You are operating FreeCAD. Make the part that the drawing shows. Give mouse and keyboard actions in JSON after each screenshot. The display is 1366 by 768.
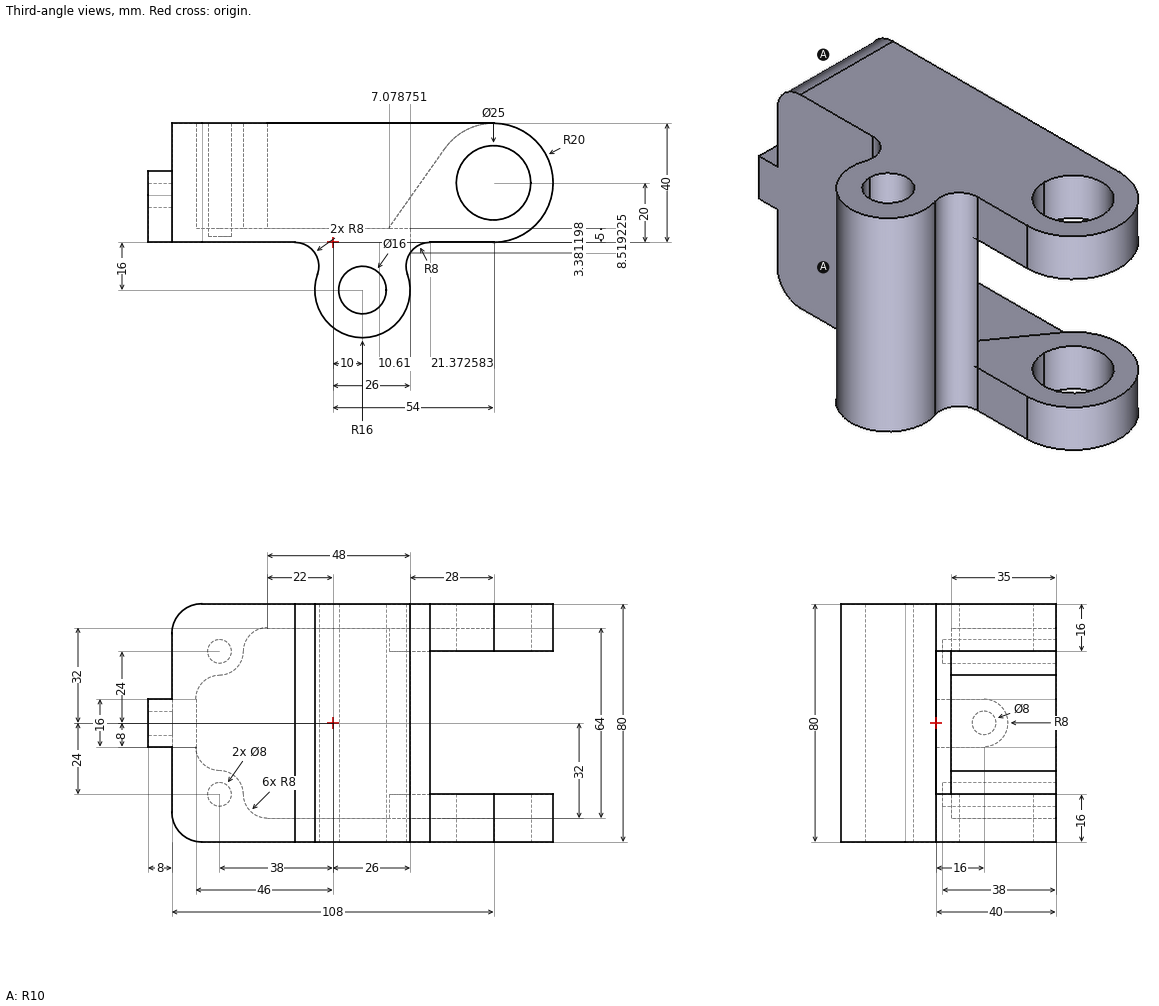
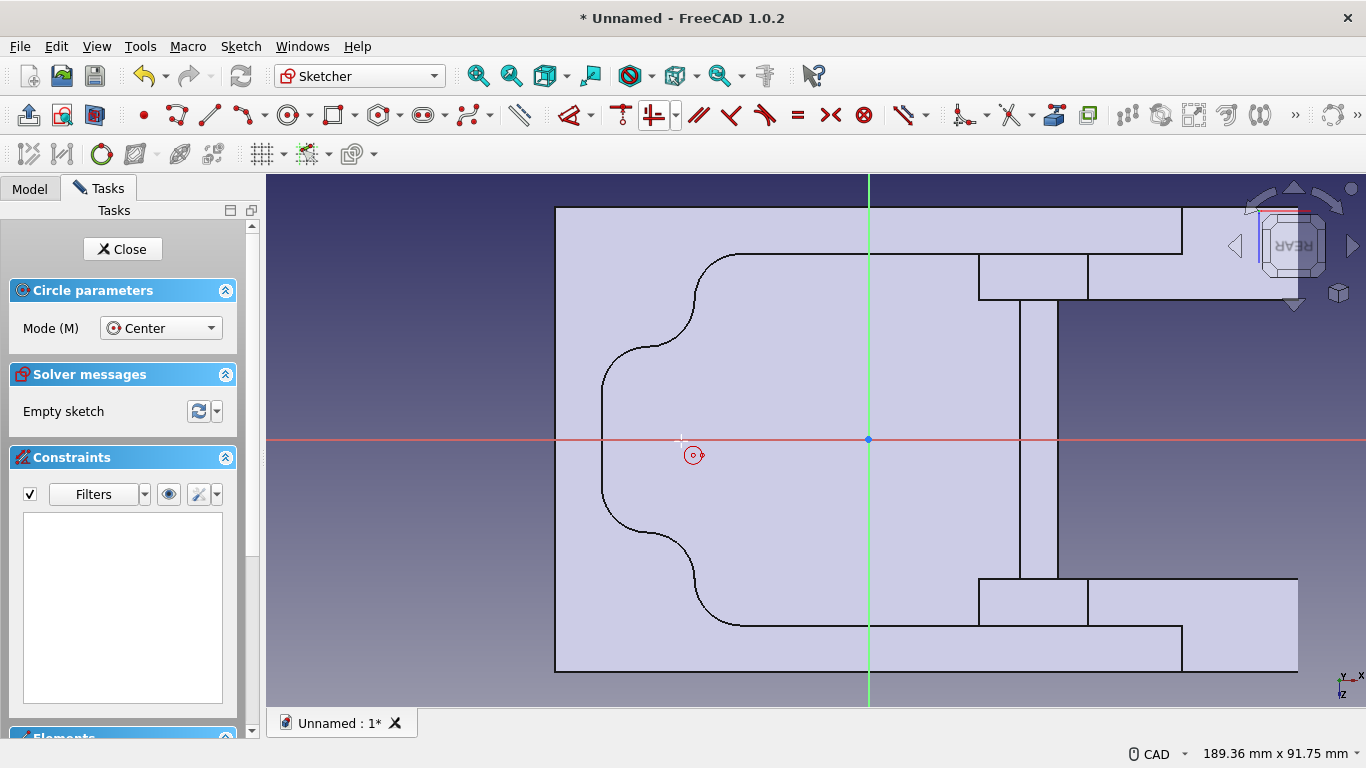
{"action": "left_click", "coordinate": [648, 300]}
{"action": "mouse_move", "coordinate": [664, 284]}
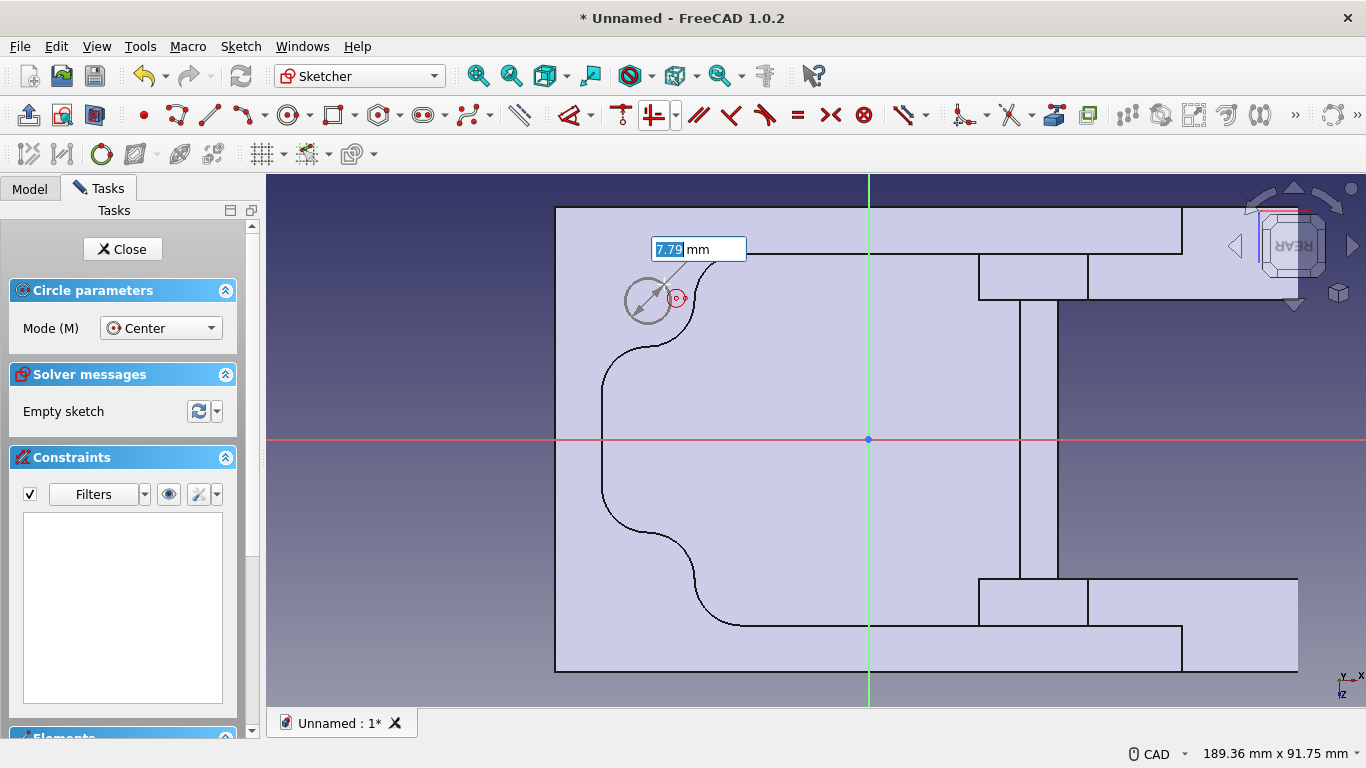
{"action": "type", "text": "8"}
{"action": "key", "text": "Return"}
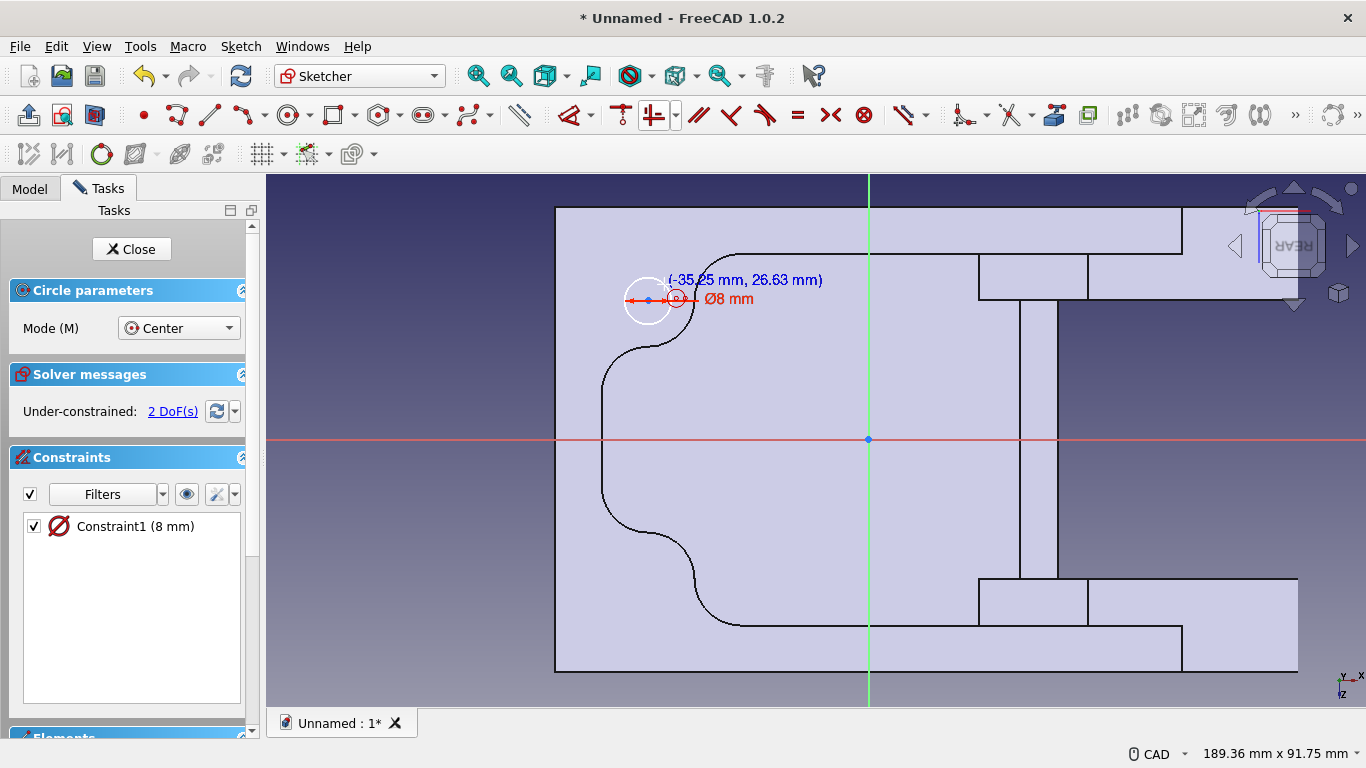
{"action": "left_click", "coordinate": [648, 579]}
{"action": "mouse_move", "coordinate": [664, 563]}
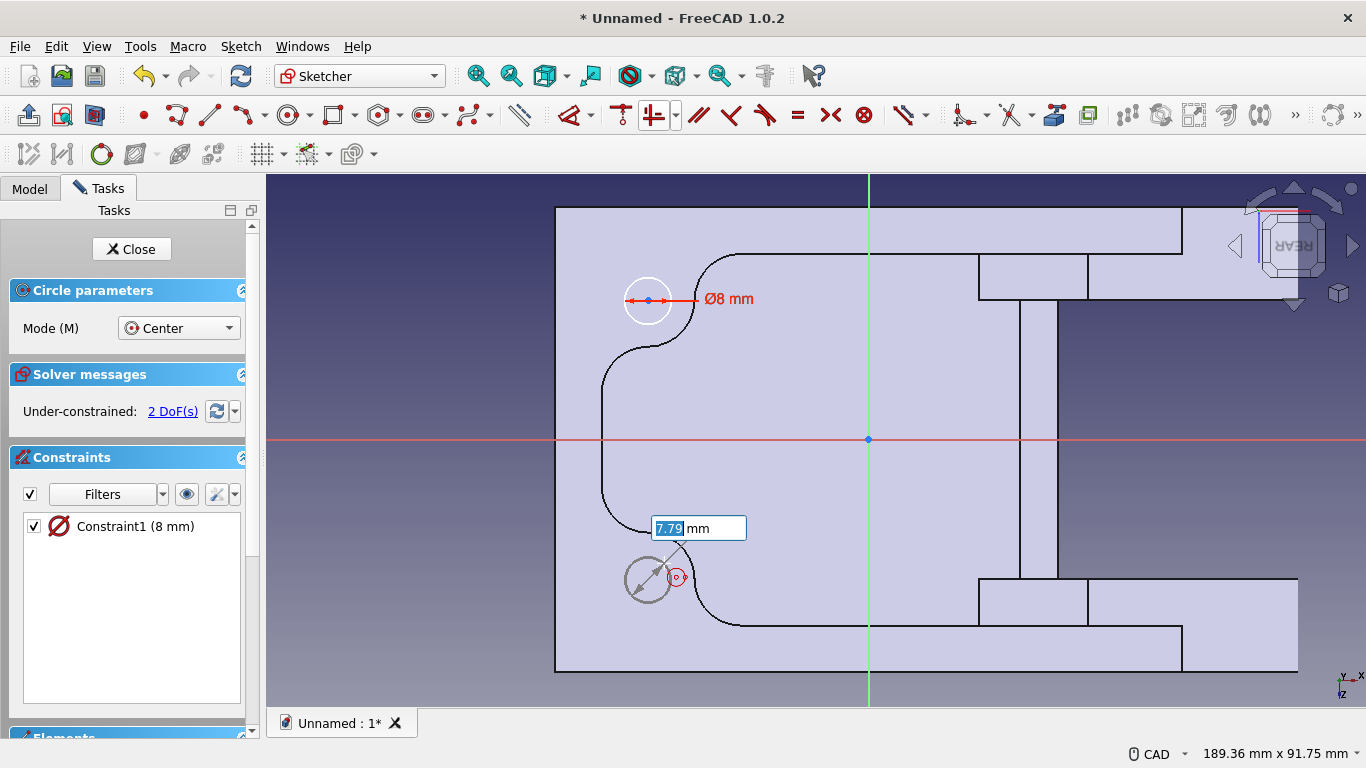
{"action": "type", "text": "8"}
{"action": "key", "text": "Return"}
{"action": "key", "text": "Escape"}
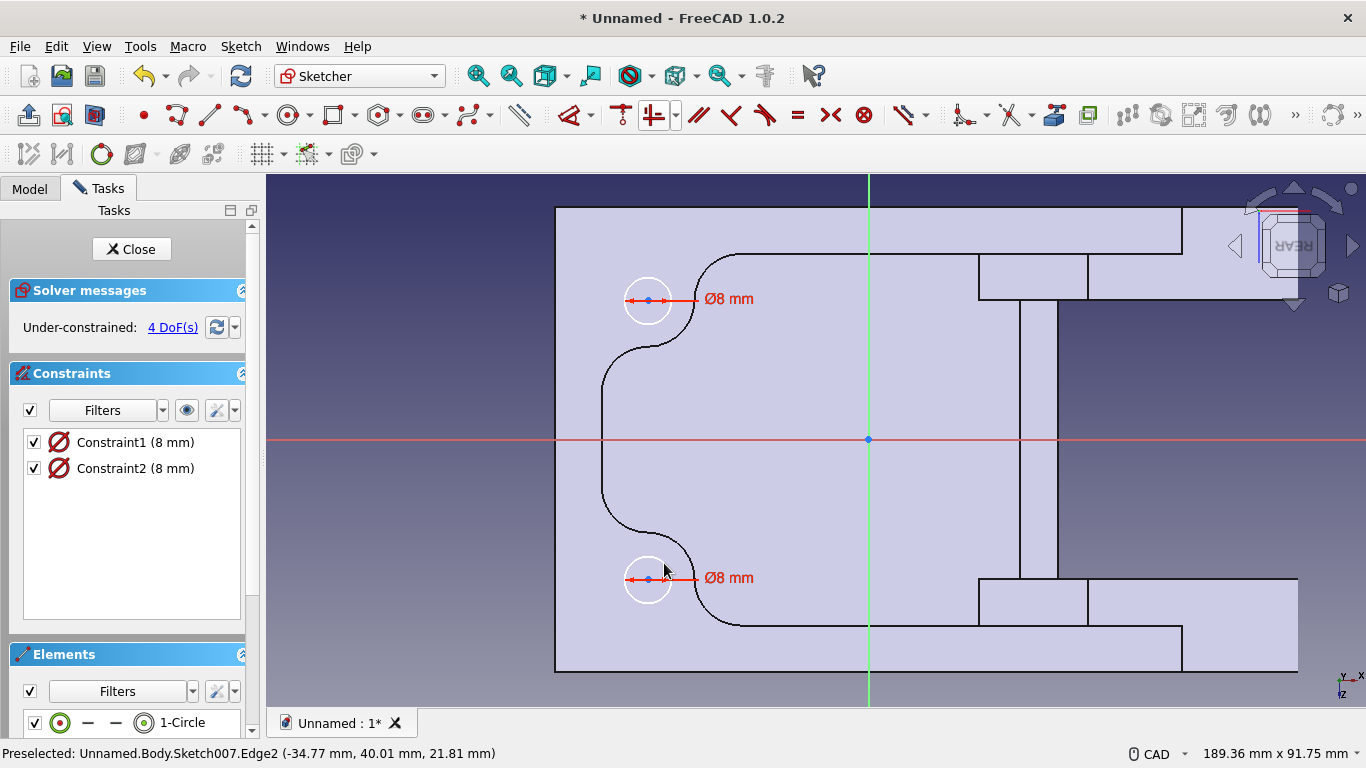
{"action": "left_click", "coordinate": [648, 301]}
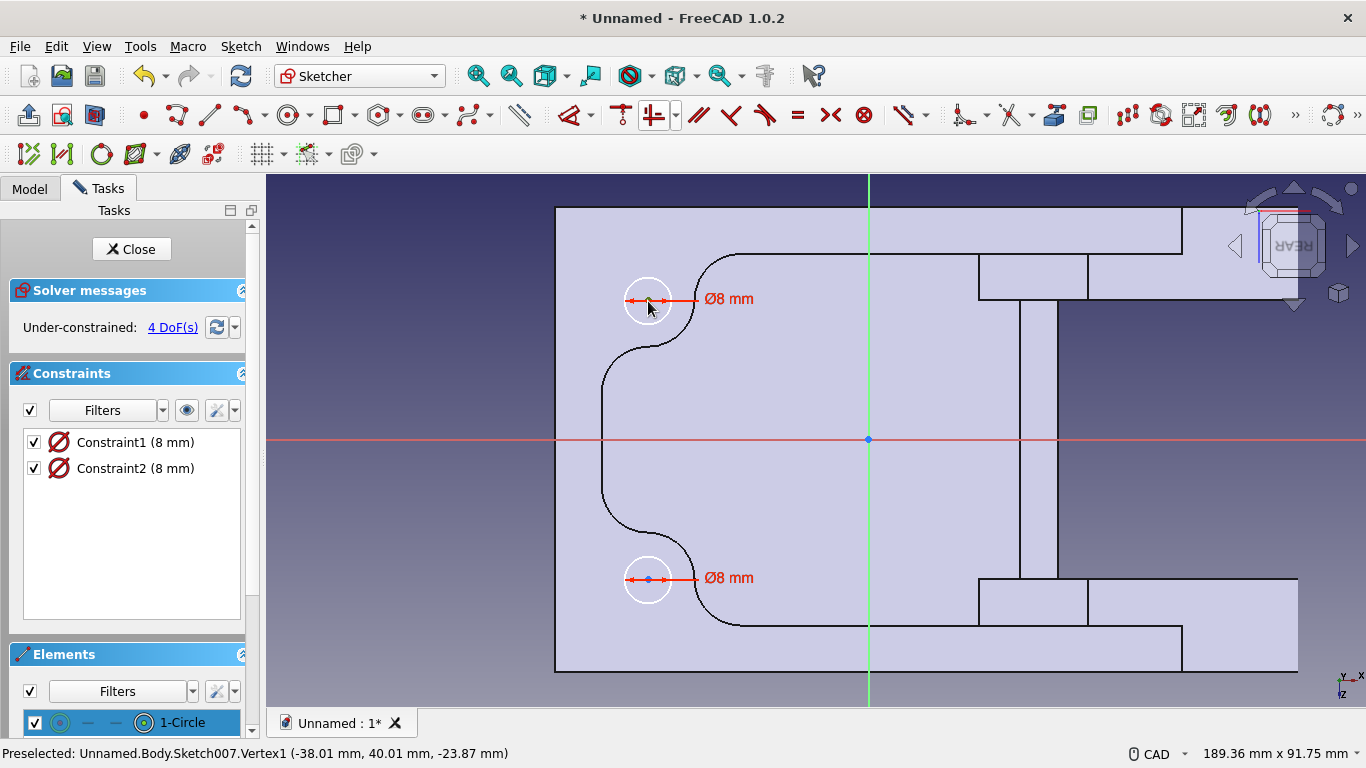
{"action": "left_click", "coordinate": [648, 580]}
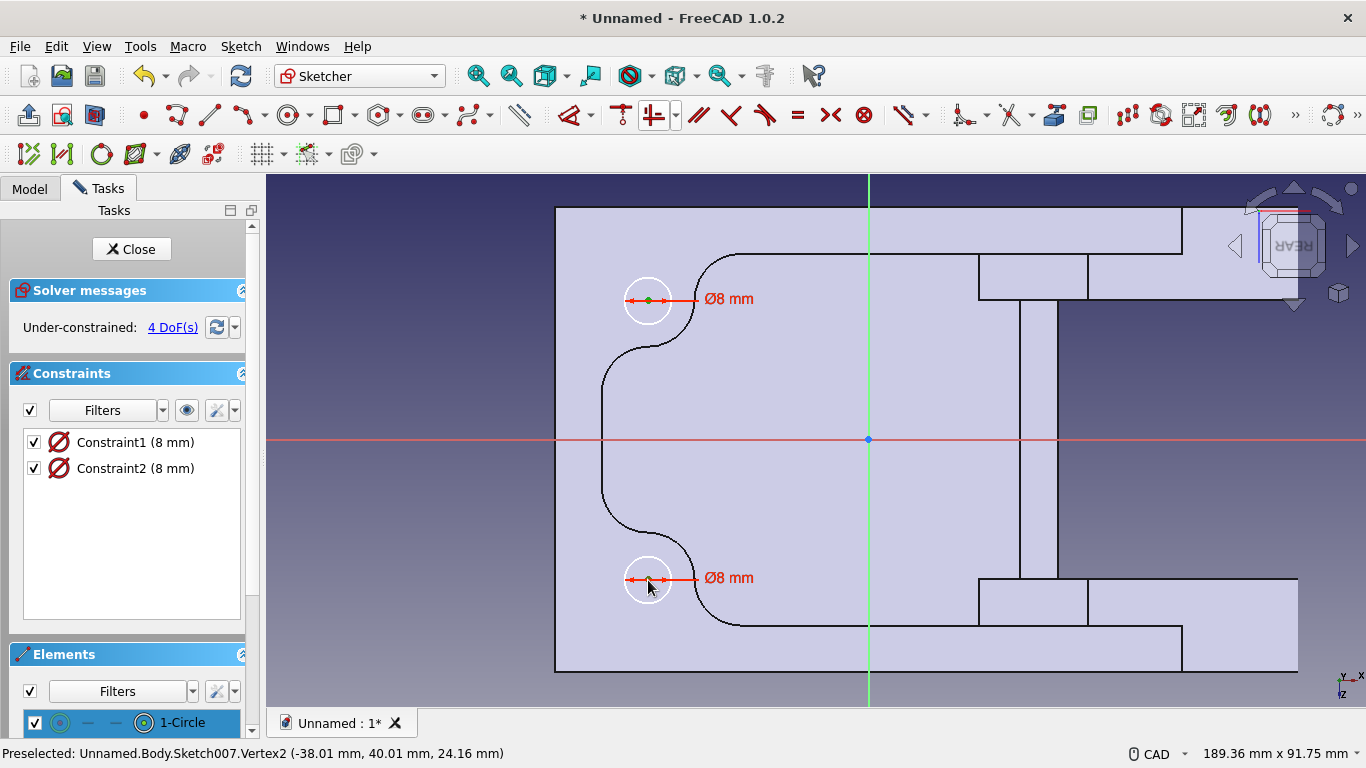
{"action": "left_click", "coordinate": [676, 116]}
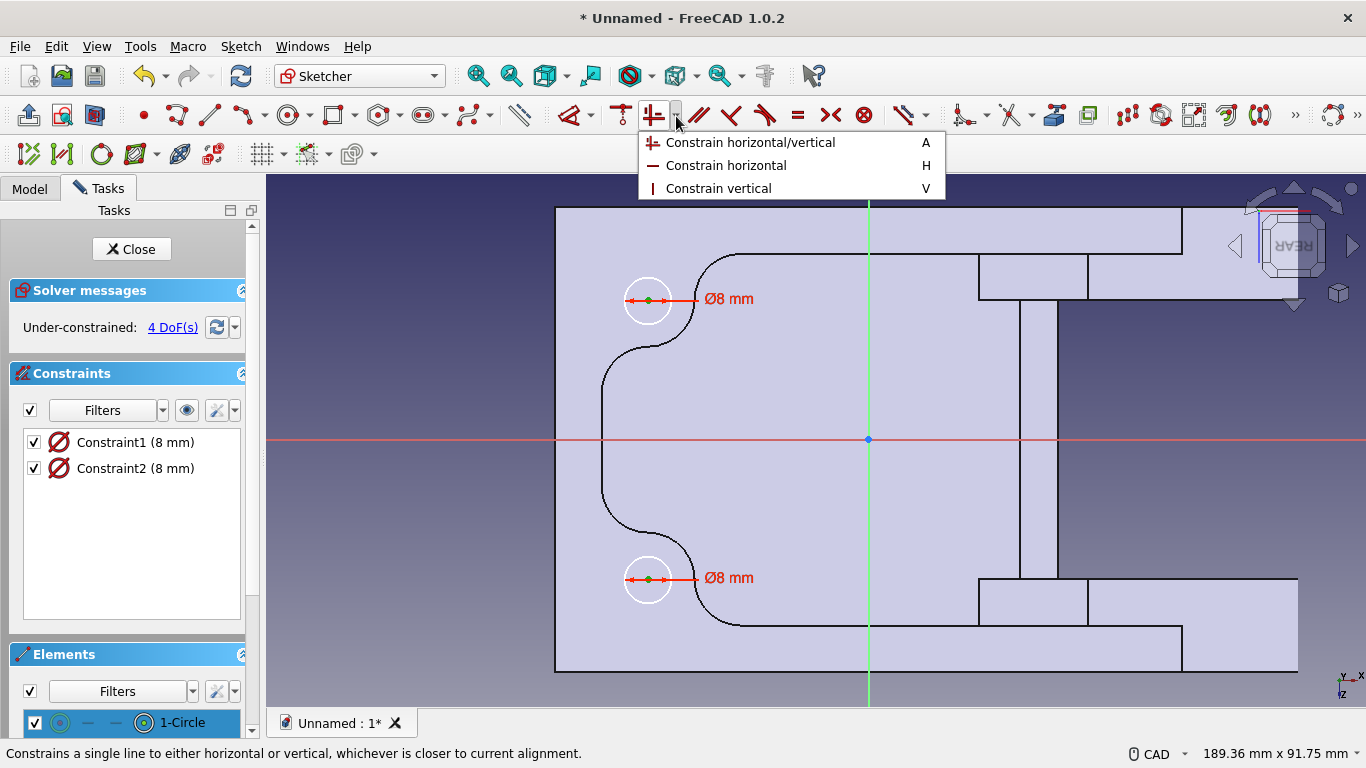
{"action": "left_click", "coordinate": [792, 188]}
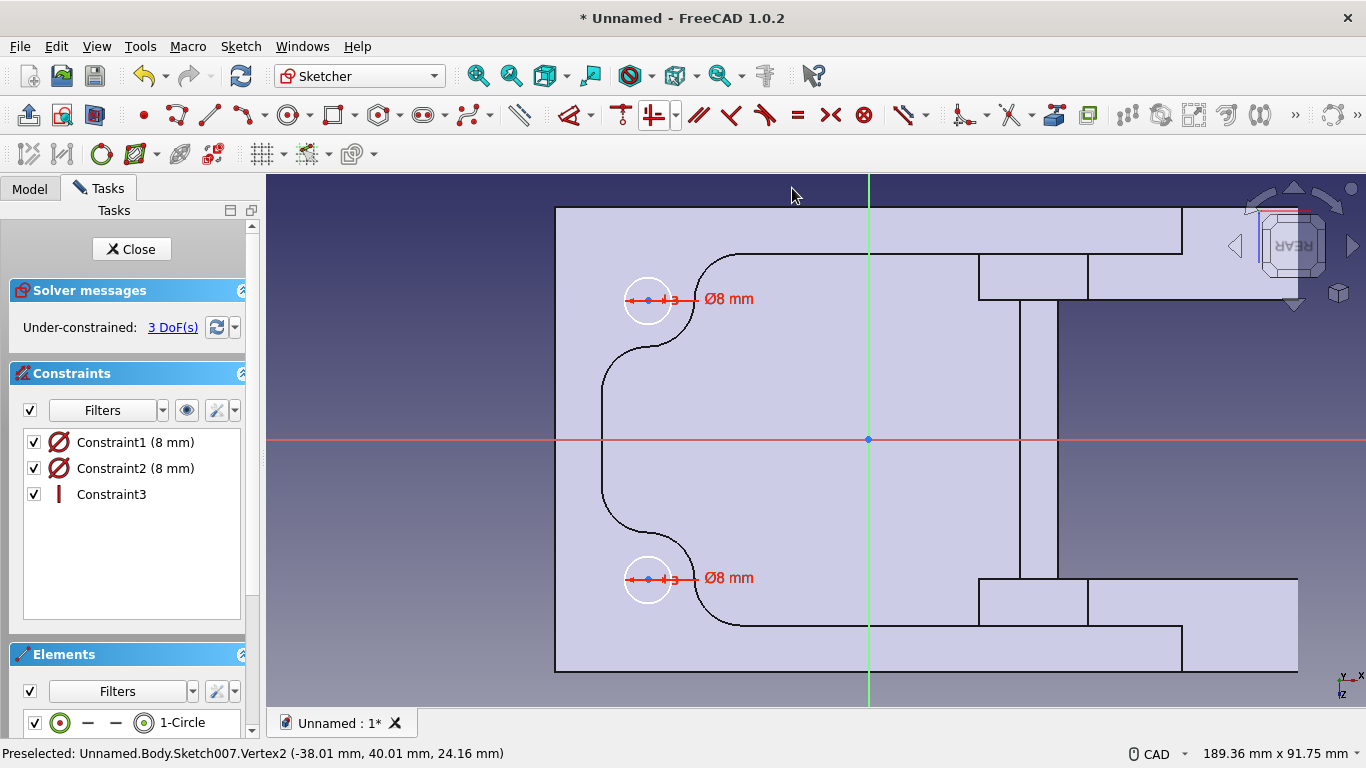
{"action": "key", "text": "d"}